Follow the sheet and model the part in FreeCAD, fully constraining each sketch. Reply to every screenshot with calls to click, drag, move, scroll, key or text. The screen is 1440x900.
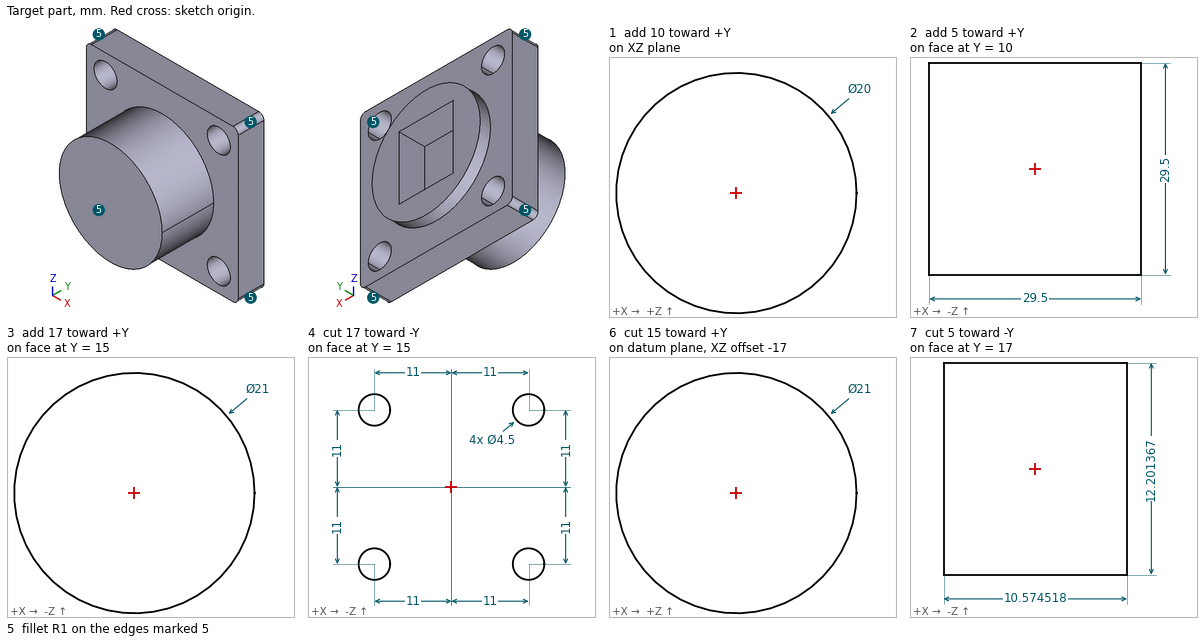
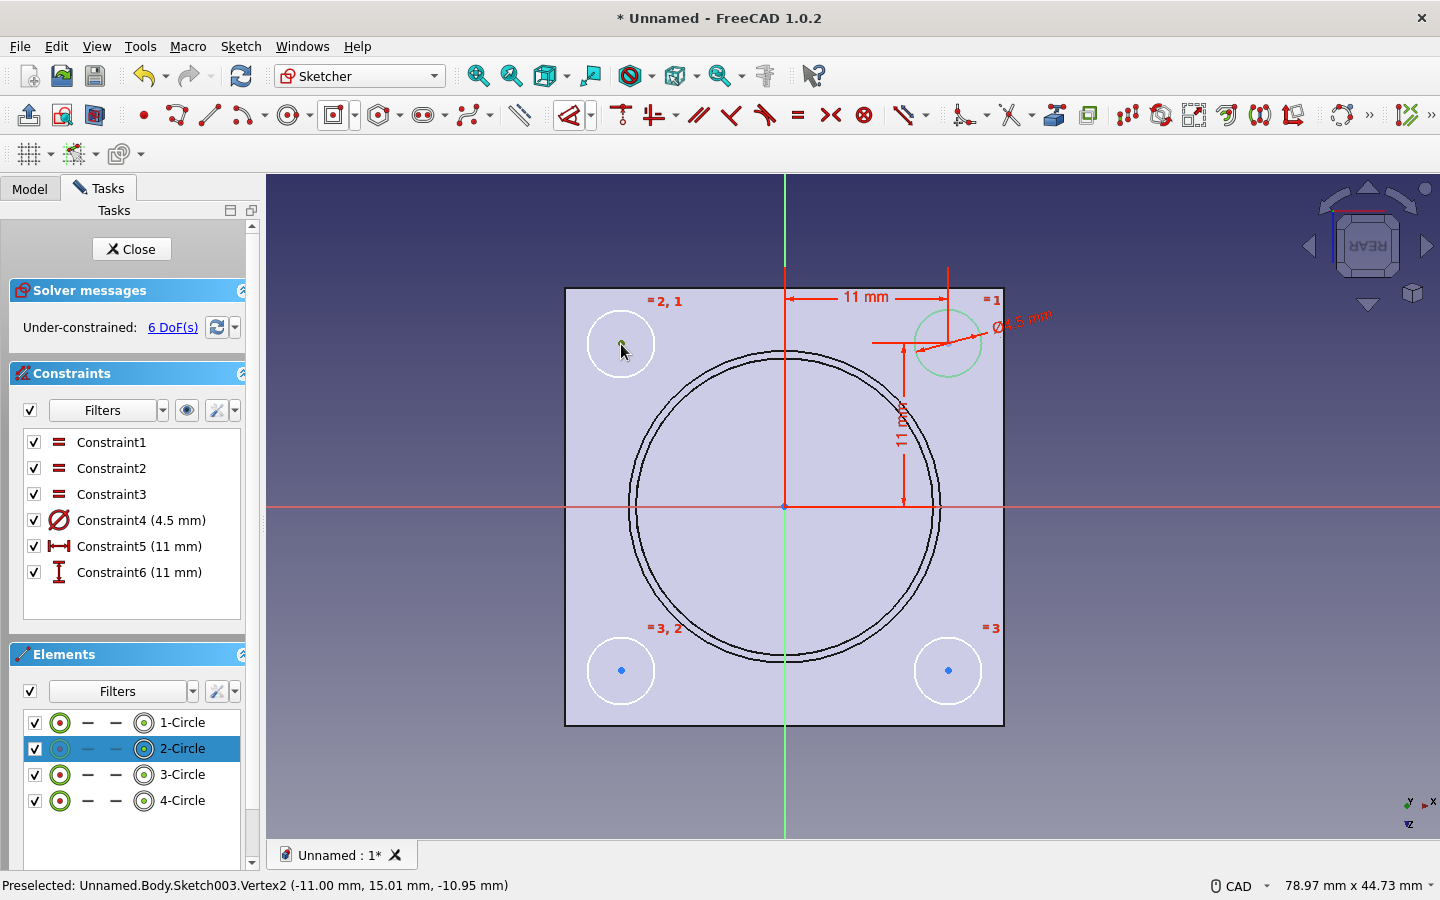
click(590, 116)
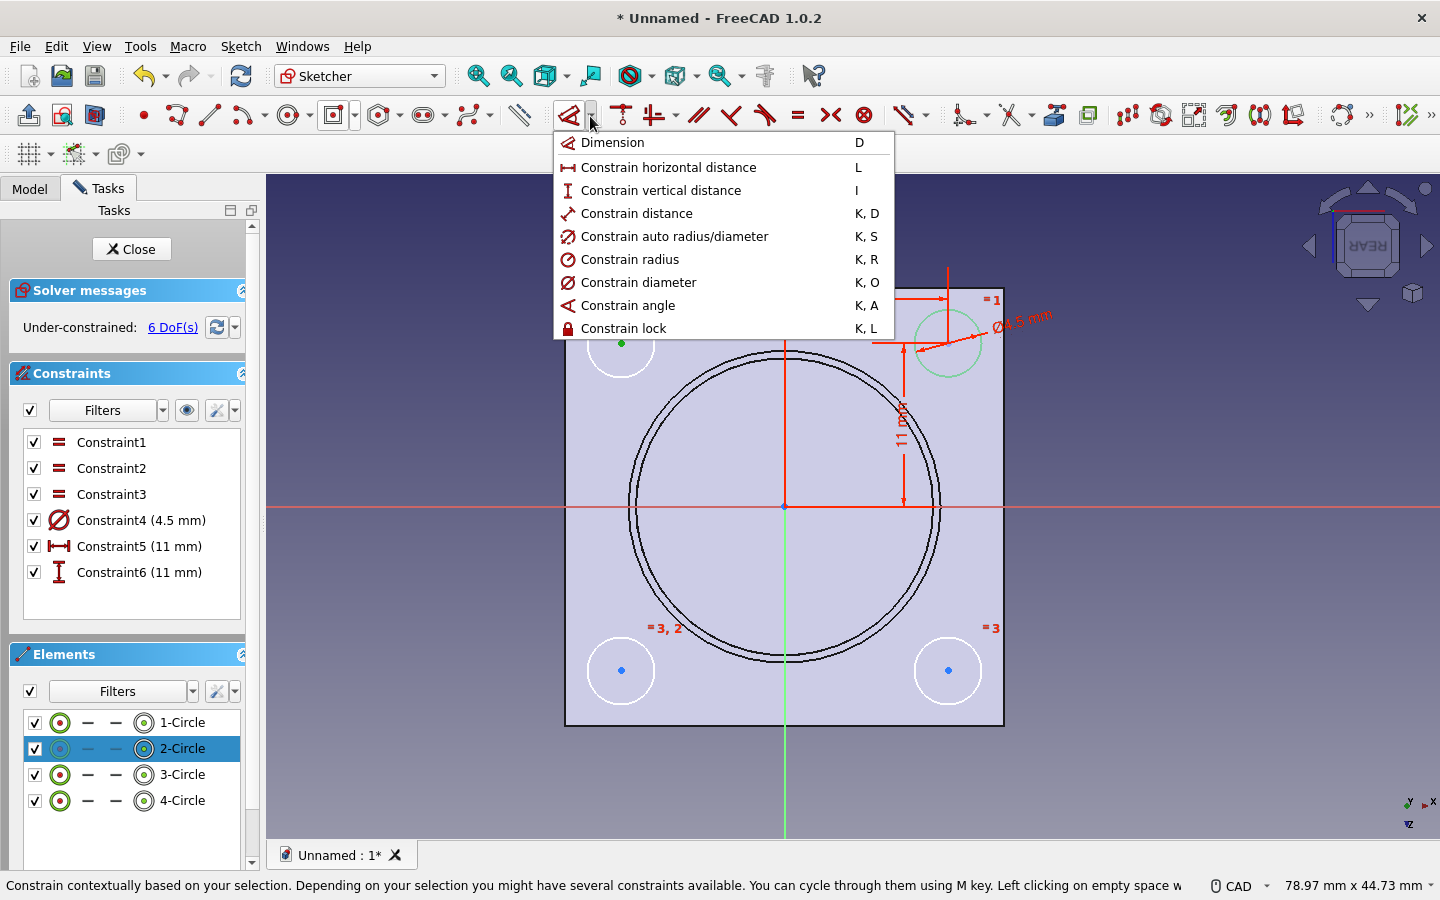
click(724, 168)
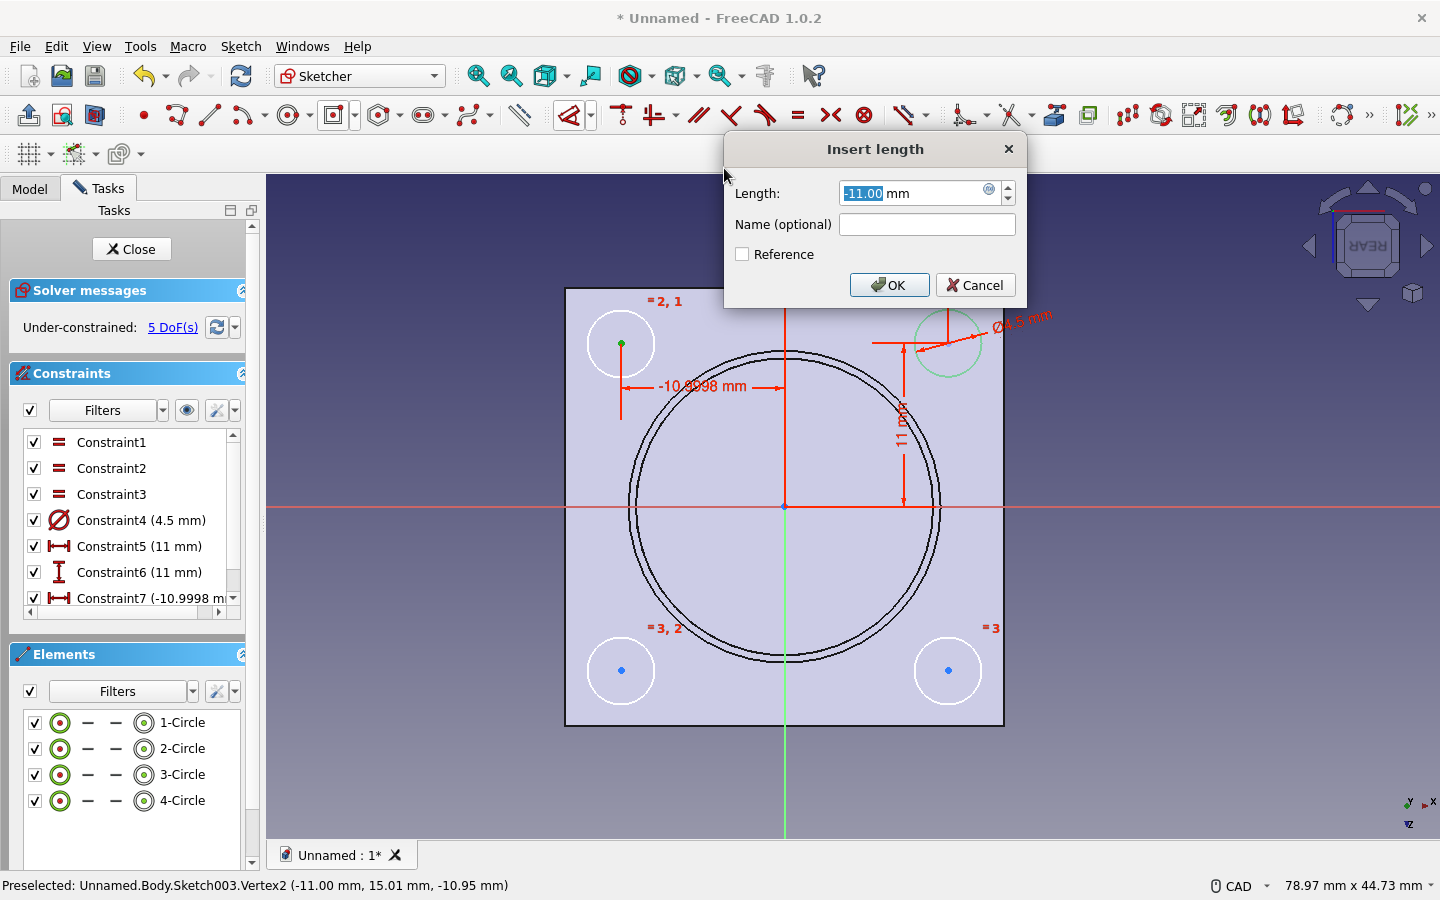
text(-11)
key(Return)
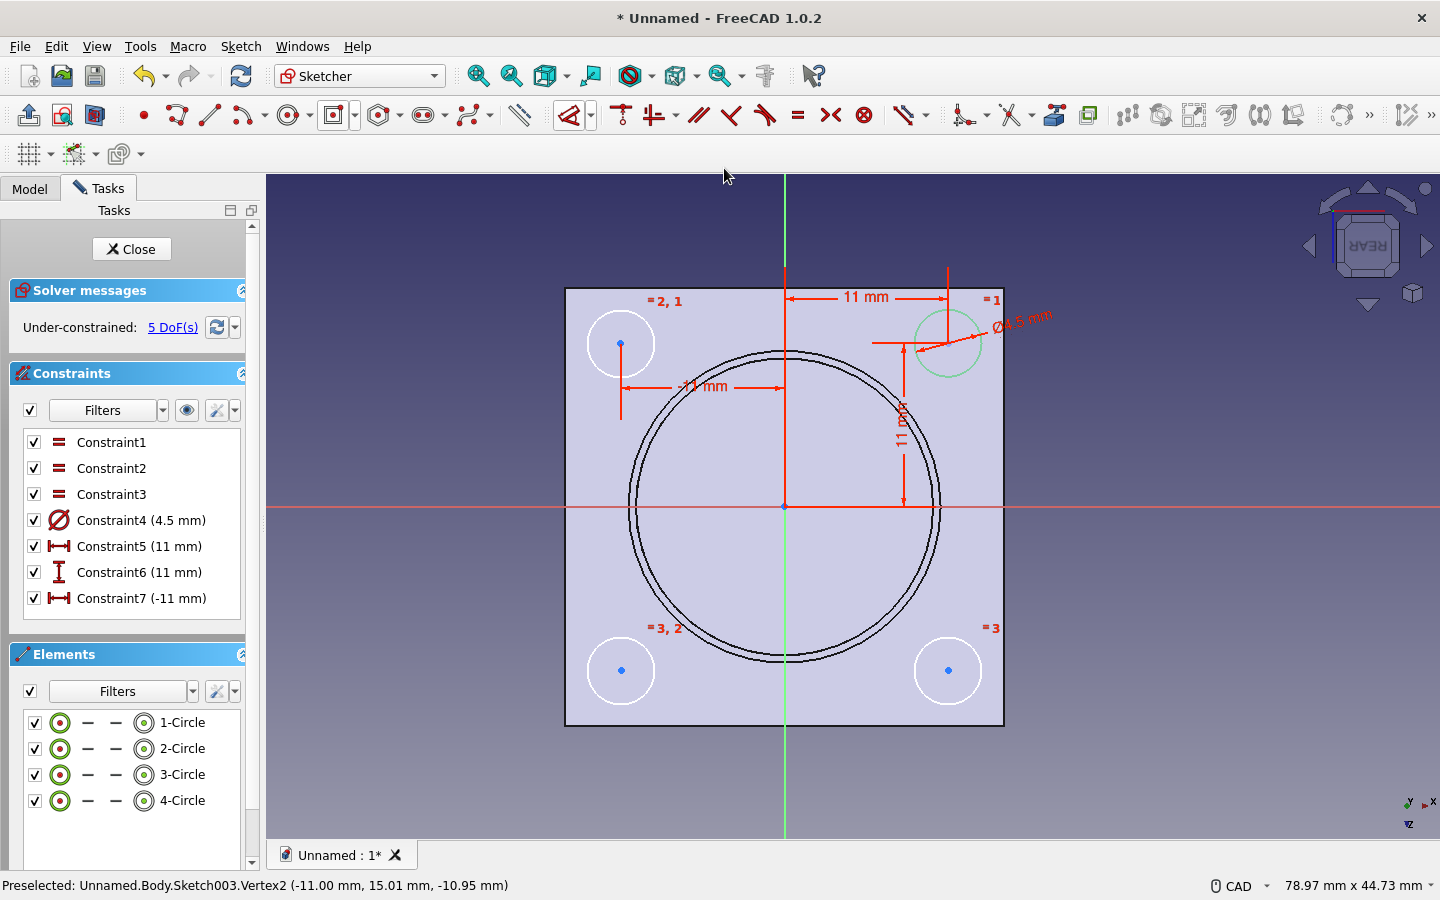
click(621, 344)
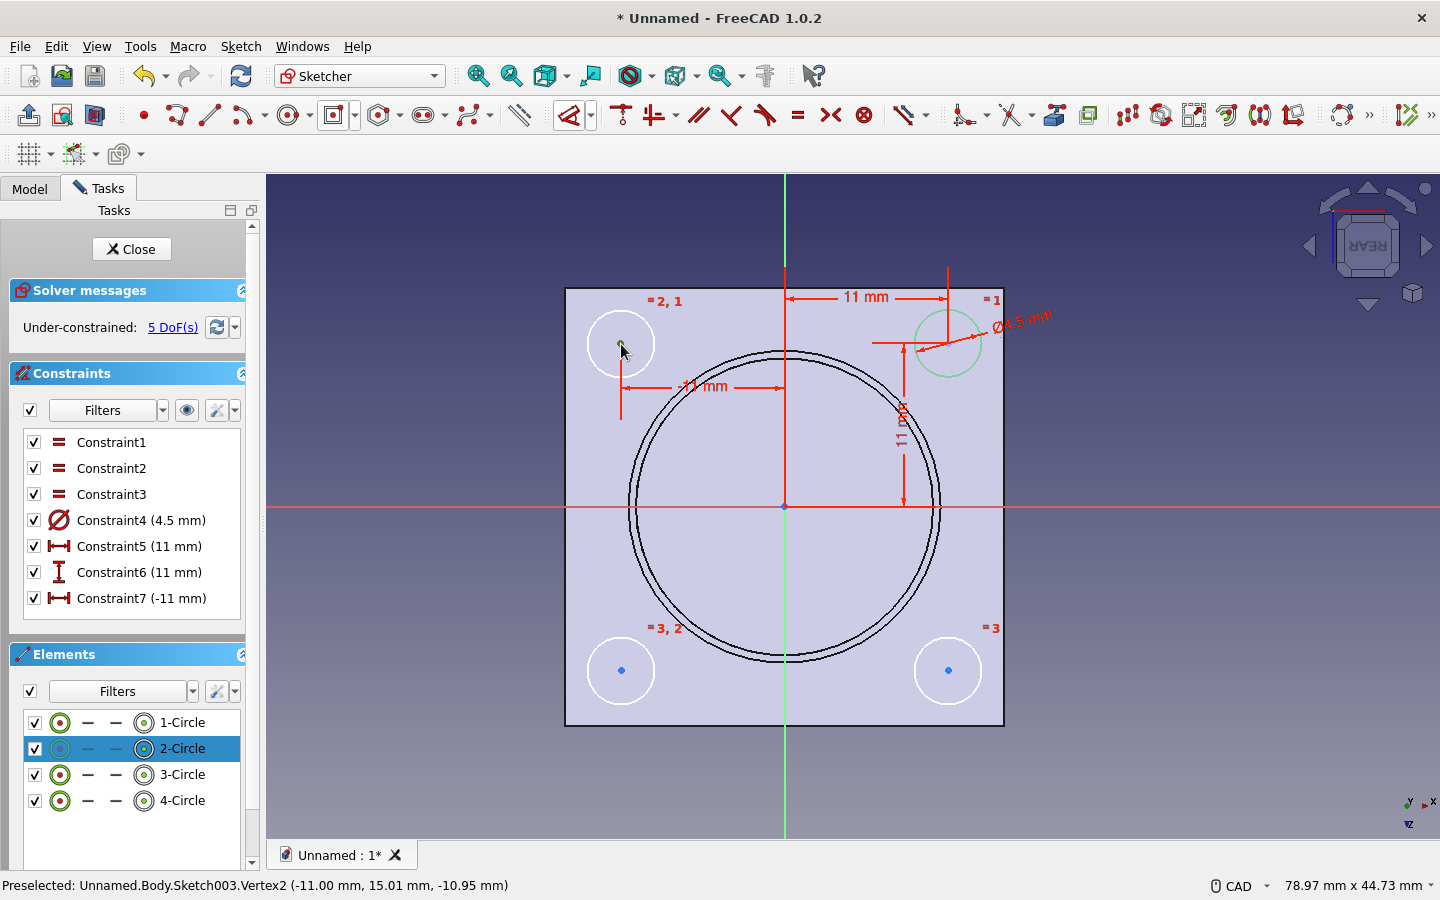
key(i)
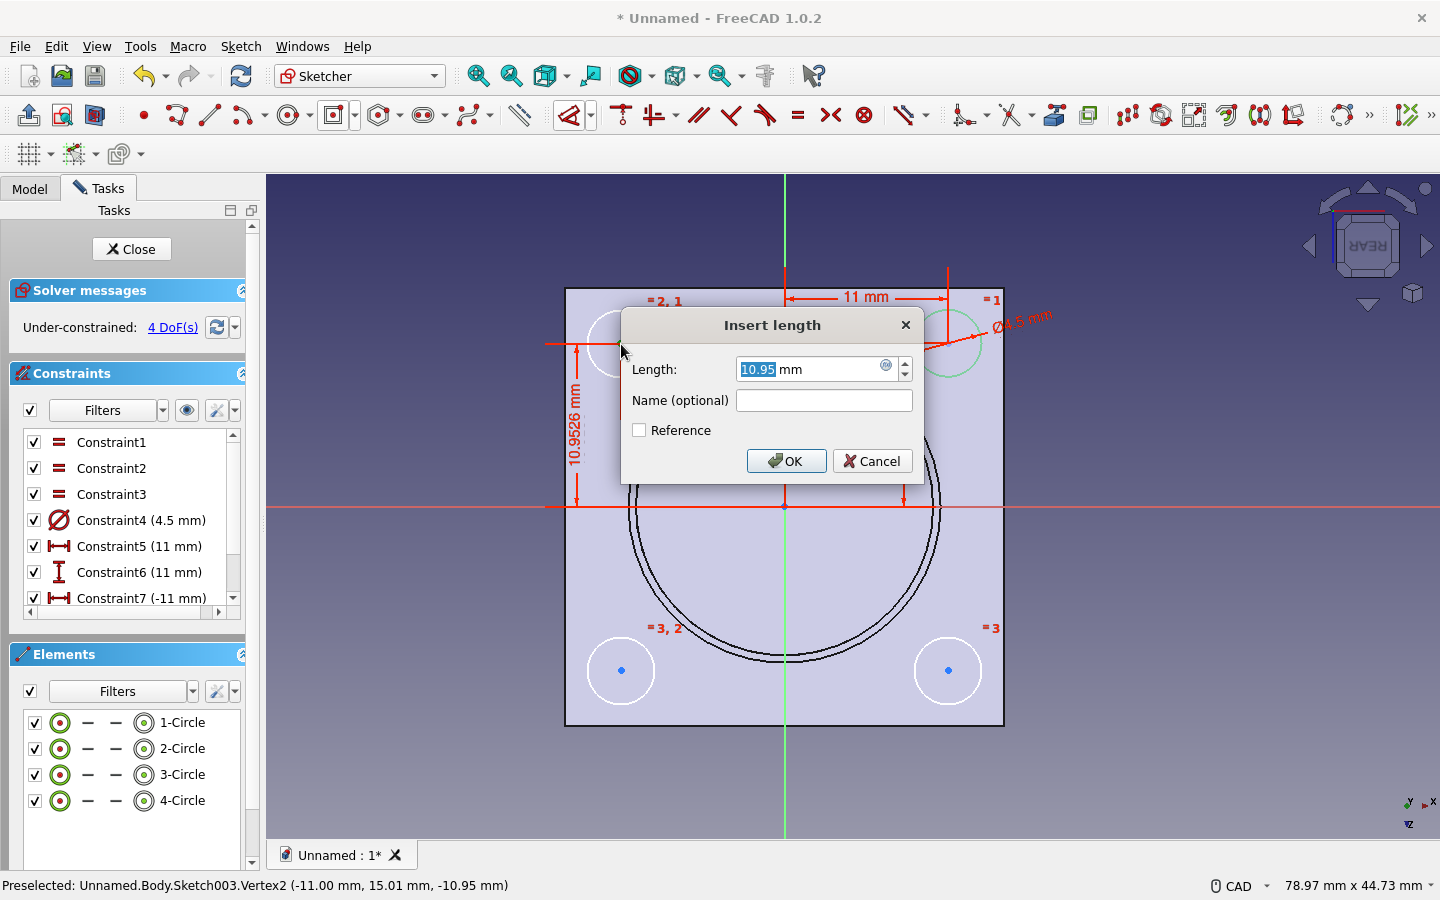
text(11)
key(Return)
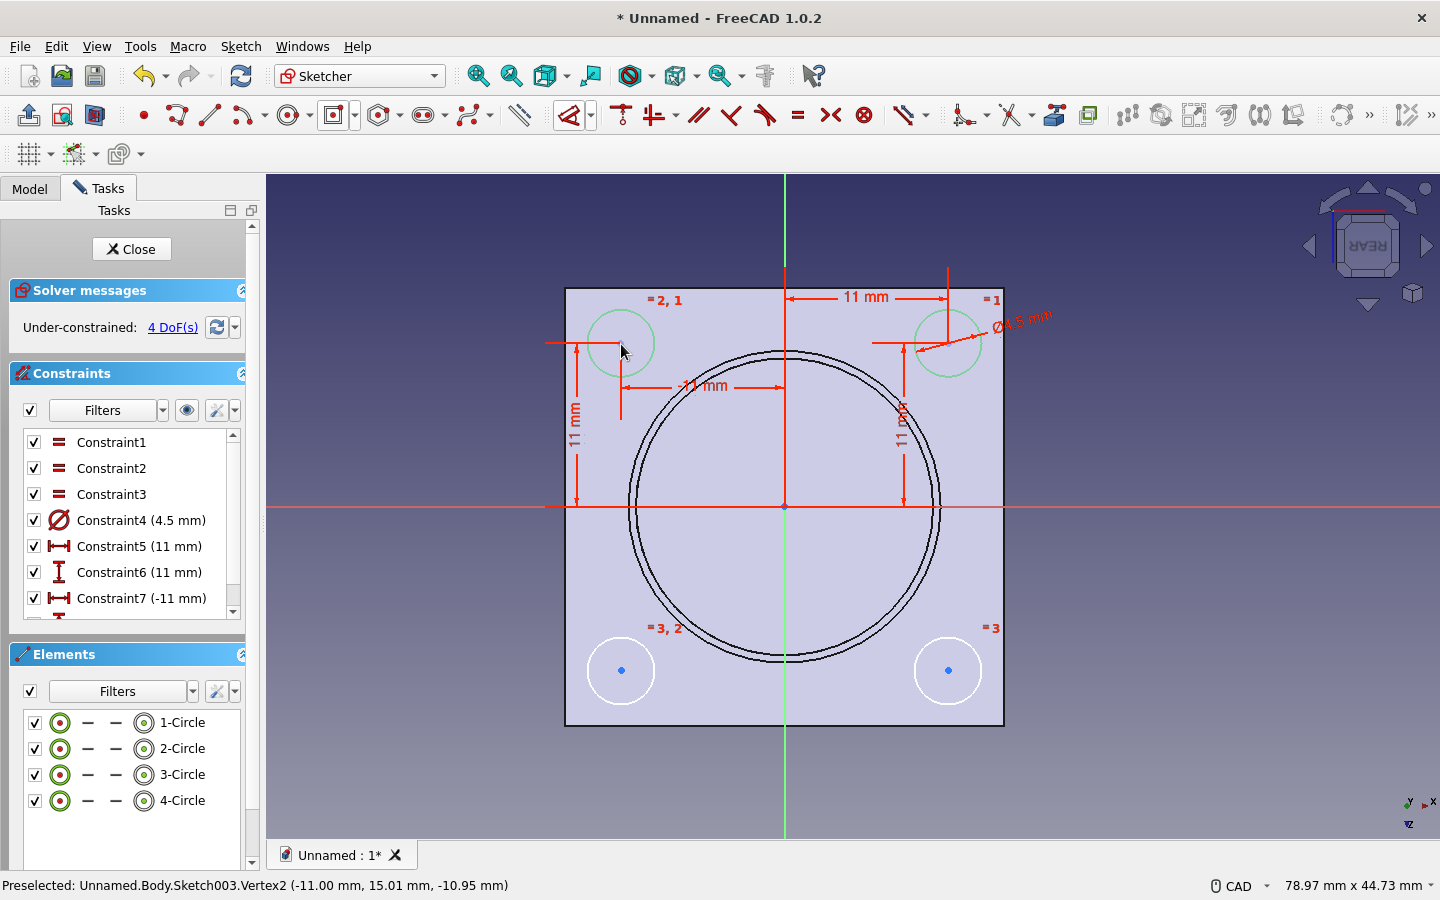
click(621, 671)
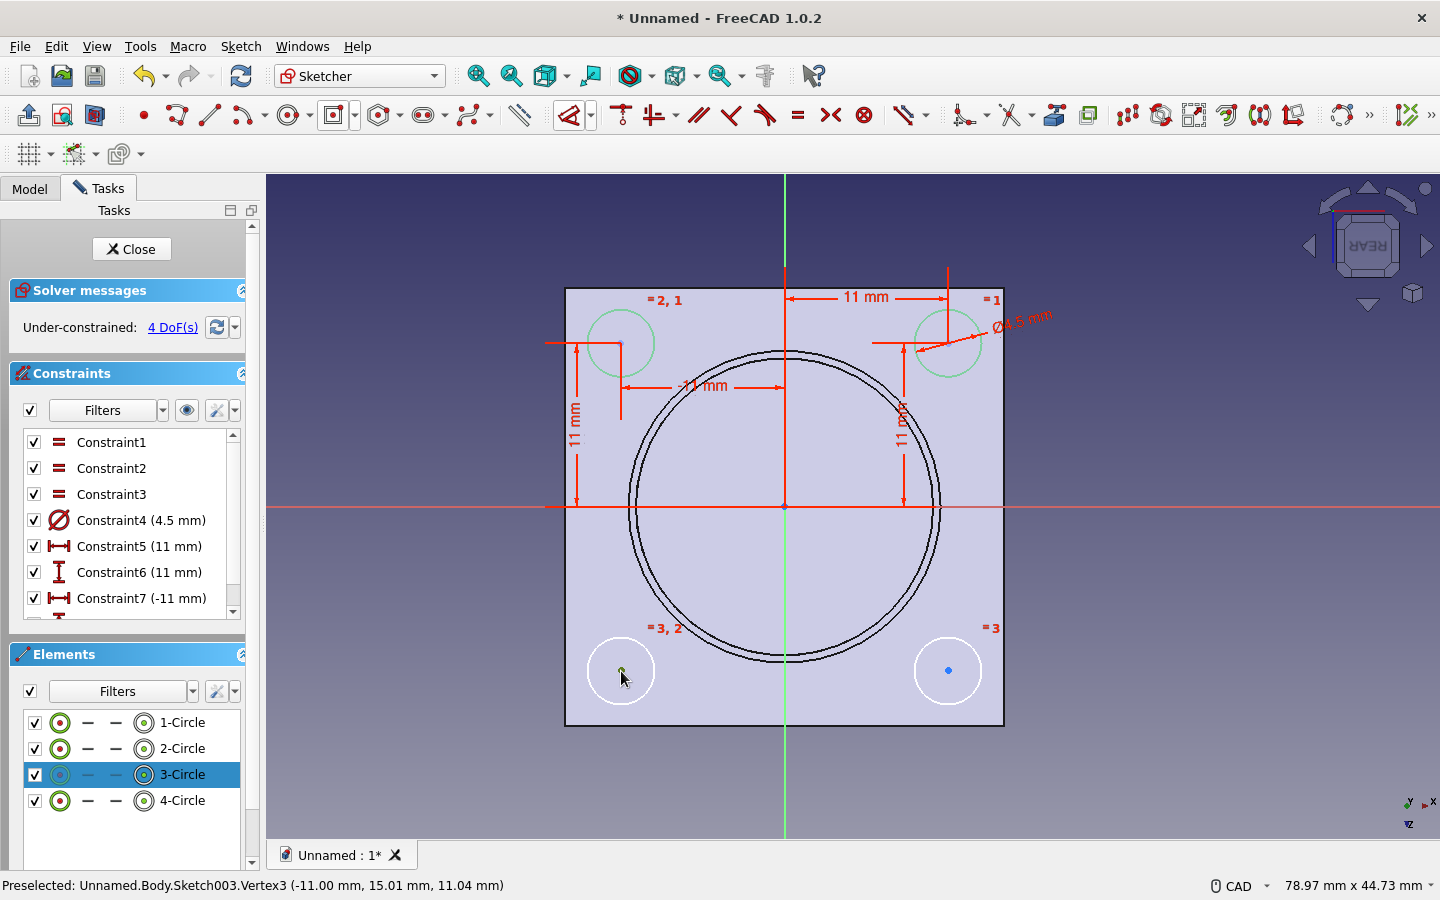
key(l)